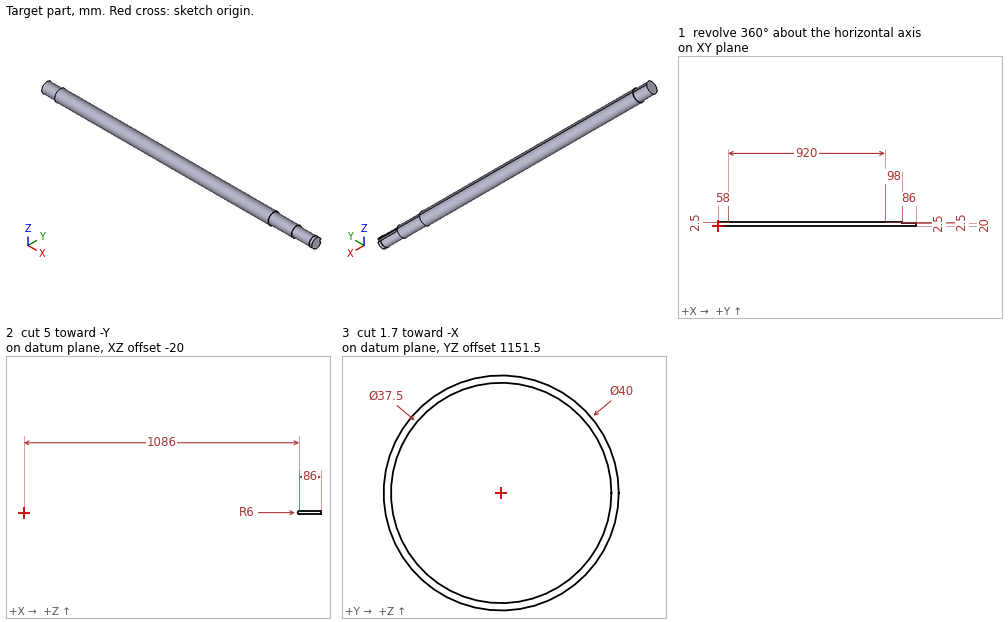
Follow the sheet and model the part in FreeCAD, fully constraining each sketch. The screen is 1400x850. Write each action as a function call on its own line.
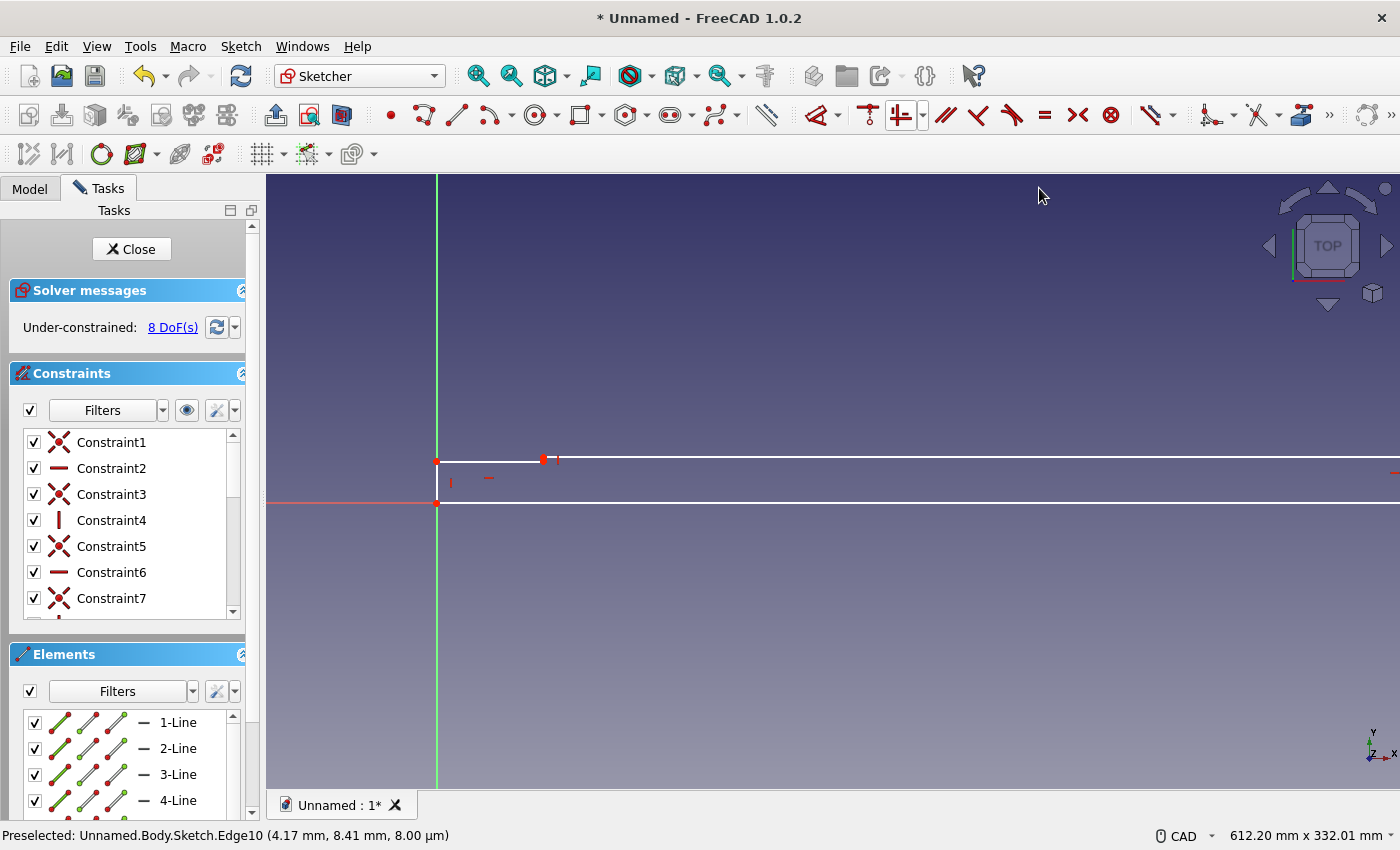
scroll(442, 482, down, 6)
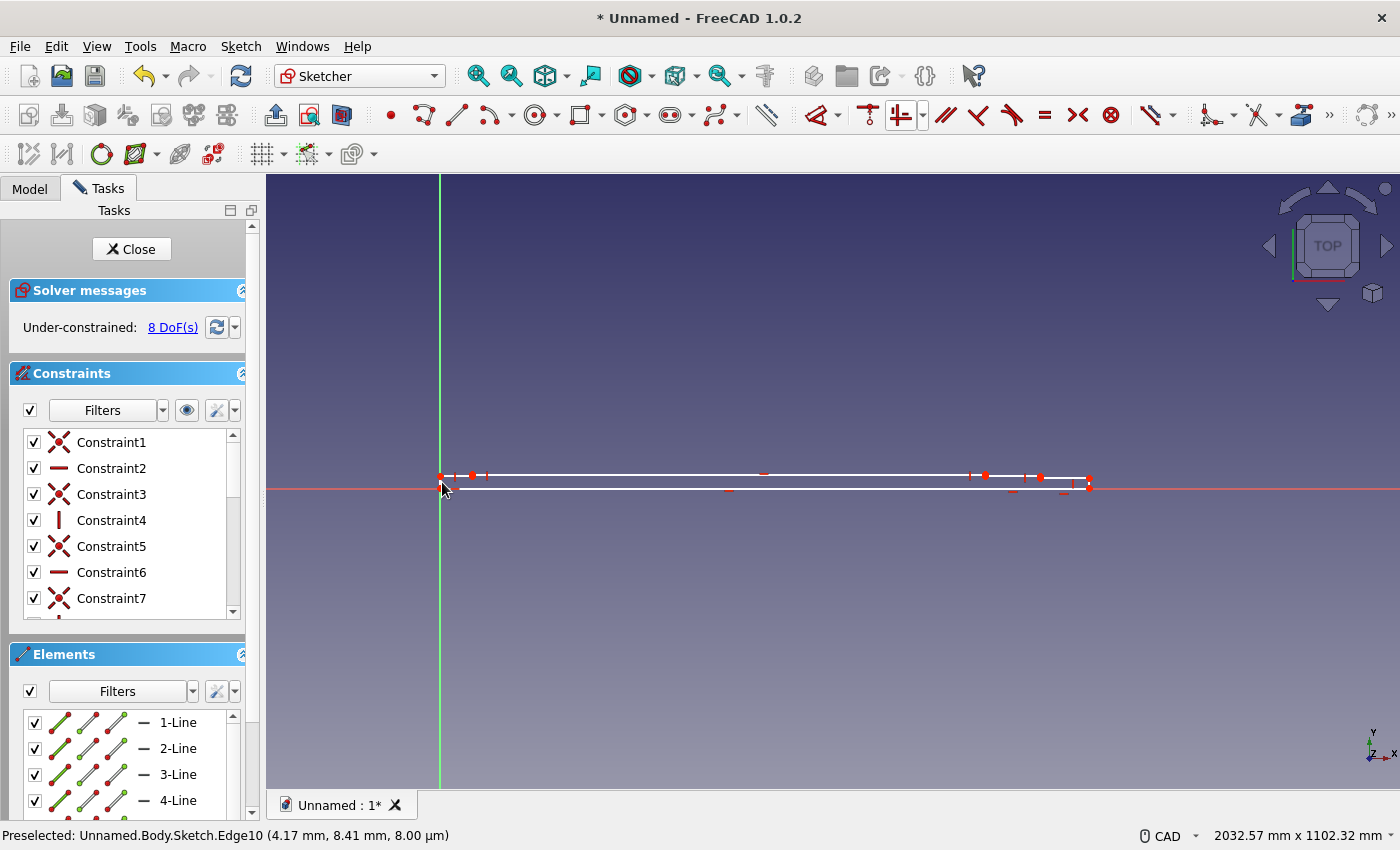
scroll(1089, 486, up, 8)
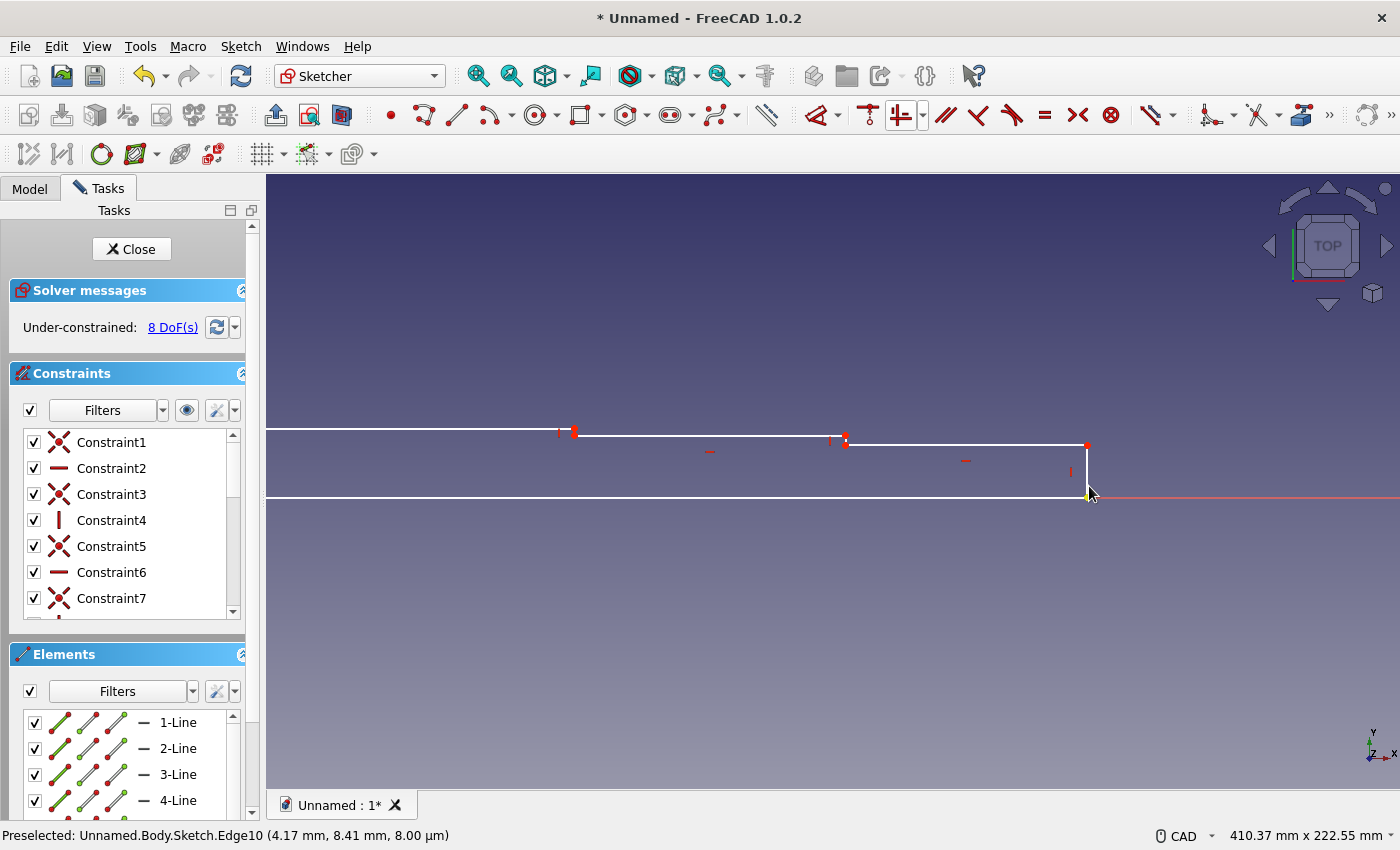
click(1087, 482)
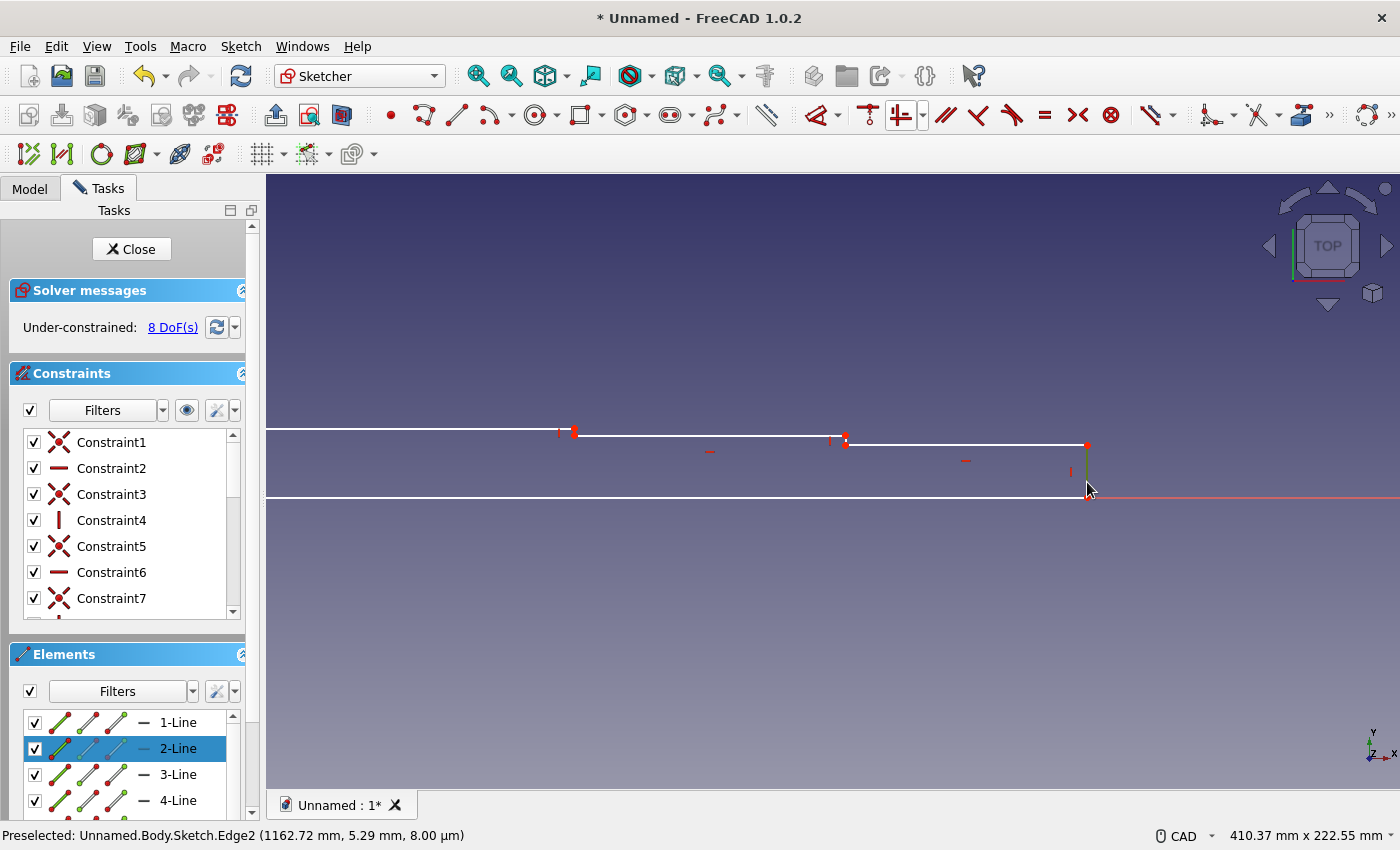
click(838, 116)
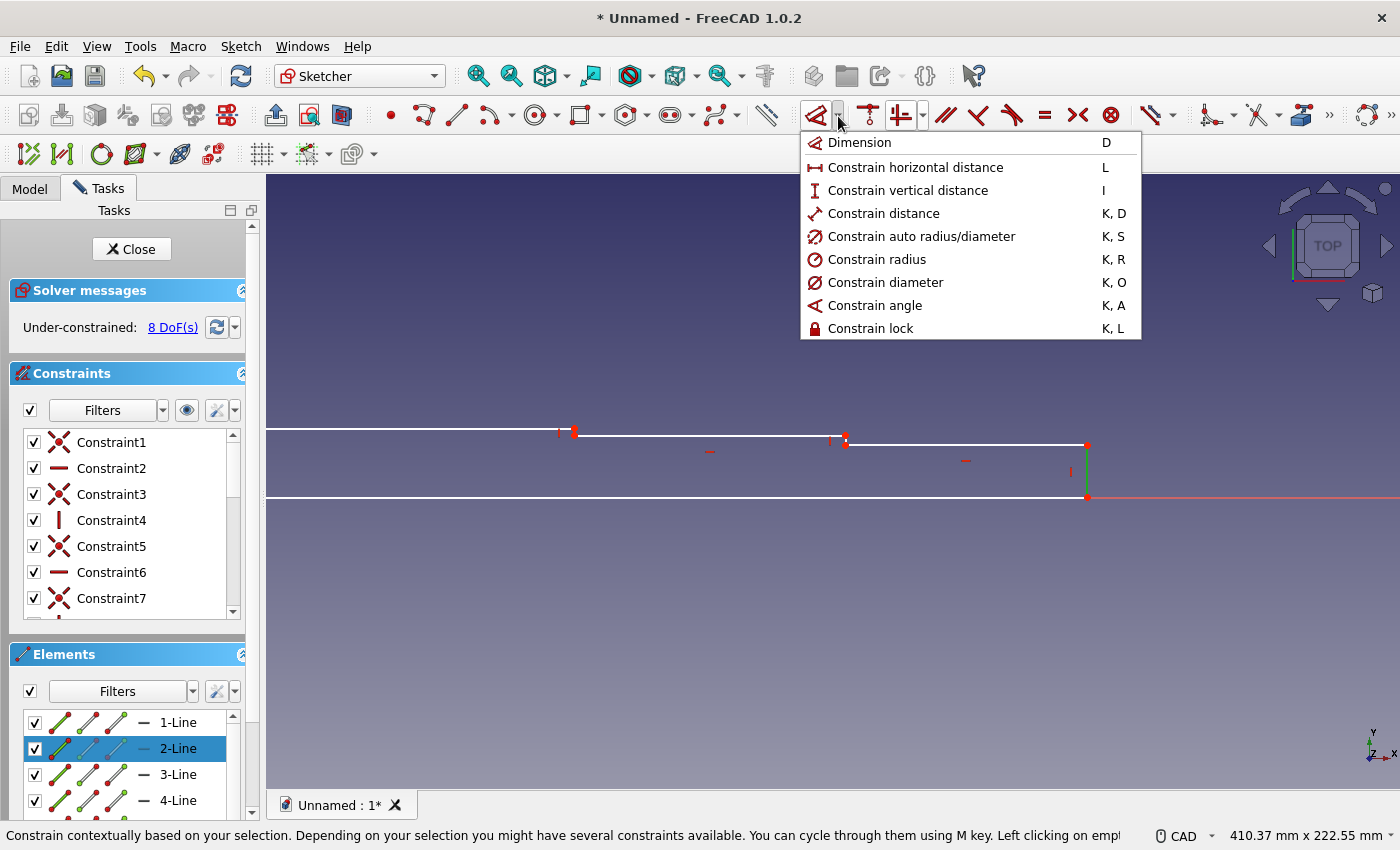
click(971, 190)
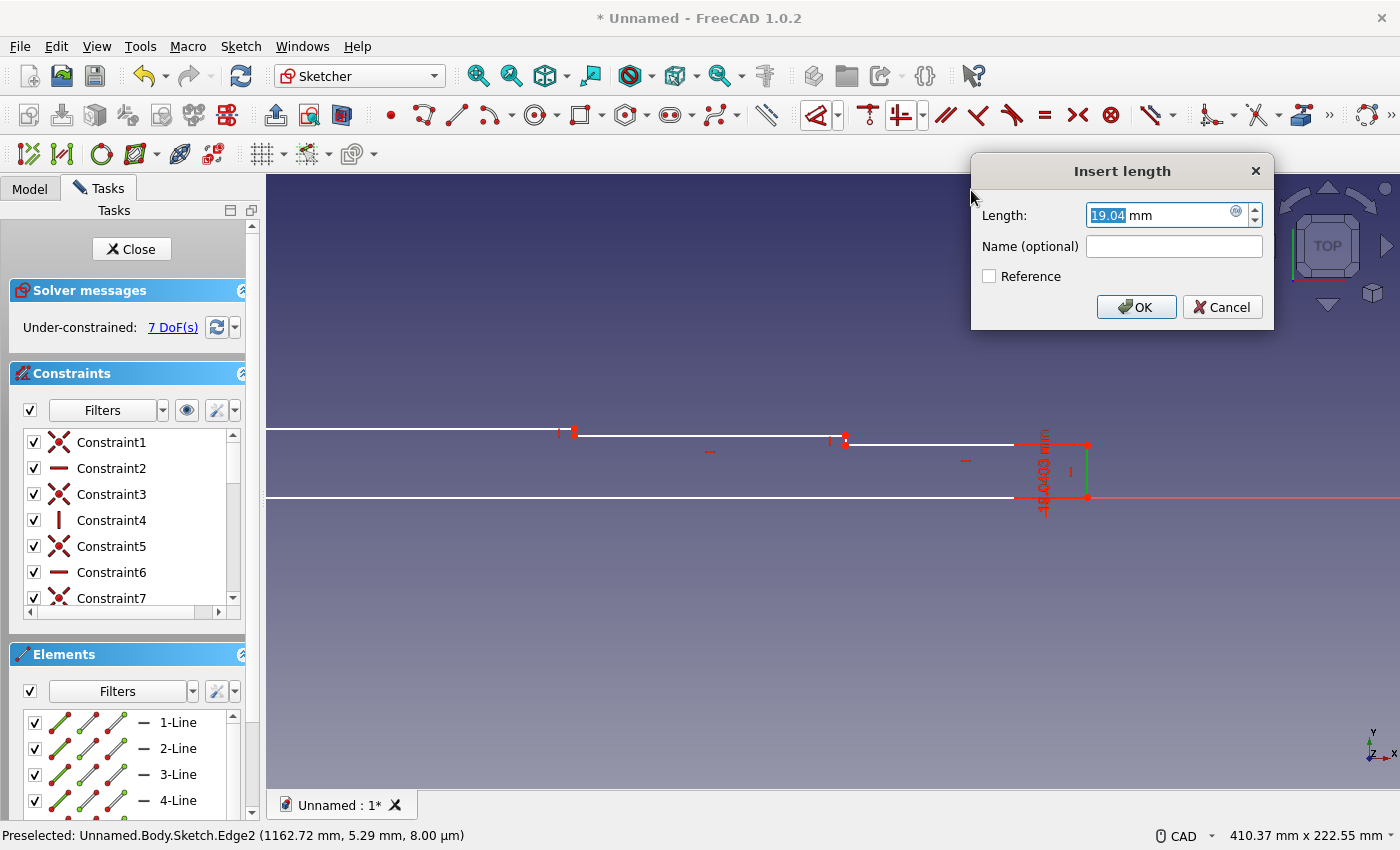
text(20)
key(Return)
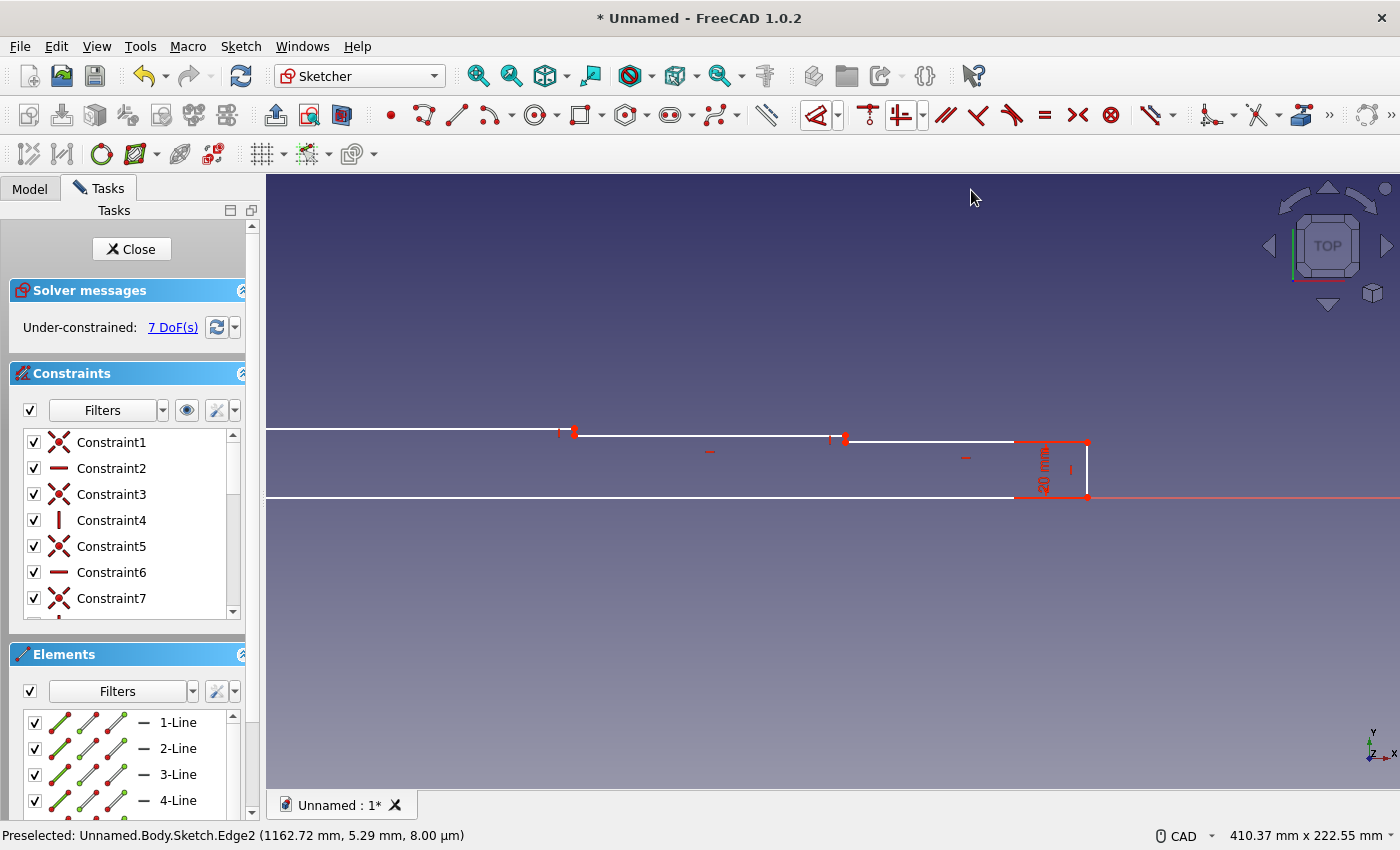
scroll(1090, 486, down, 8)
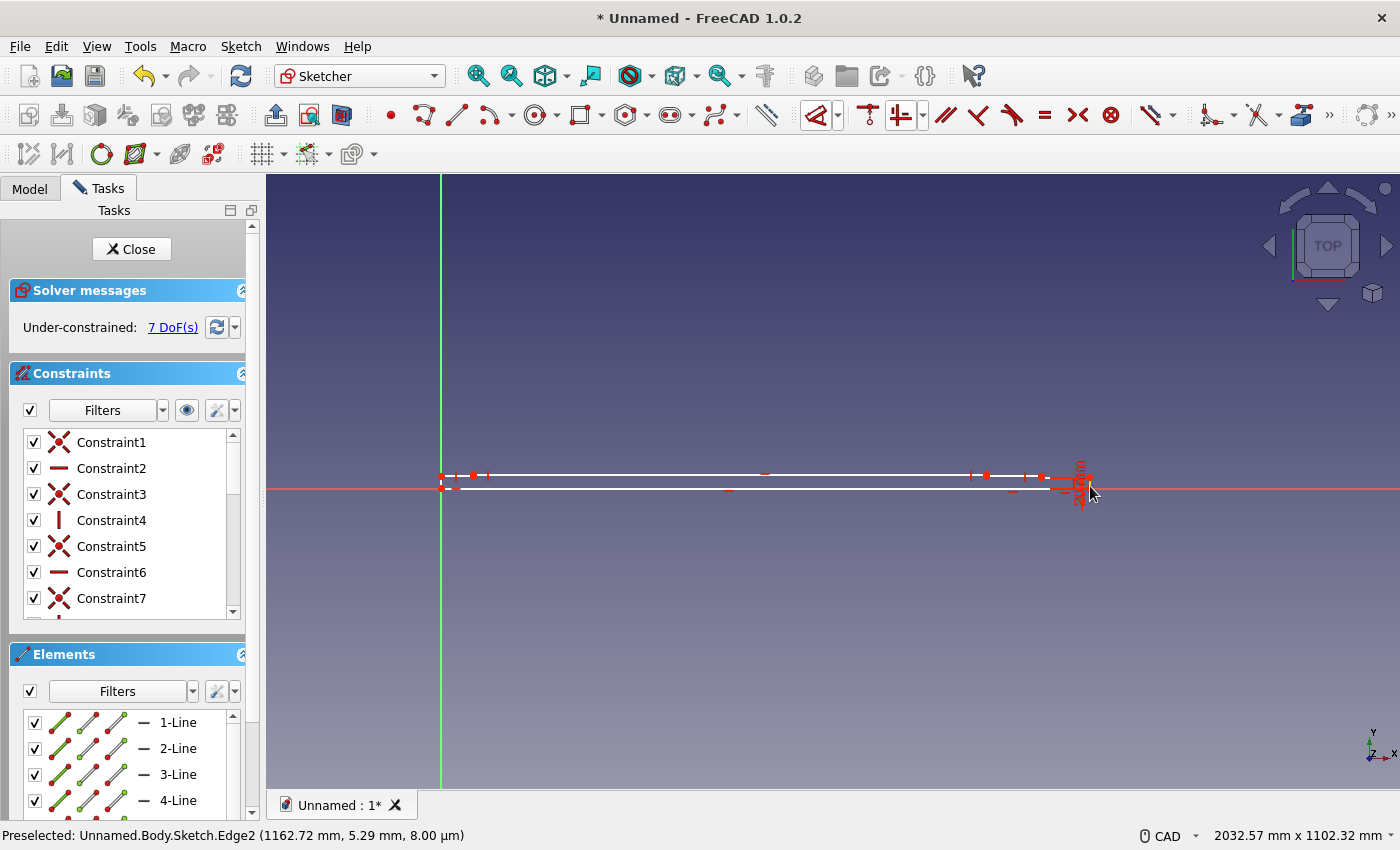
scroll(1075, 478, up, 2)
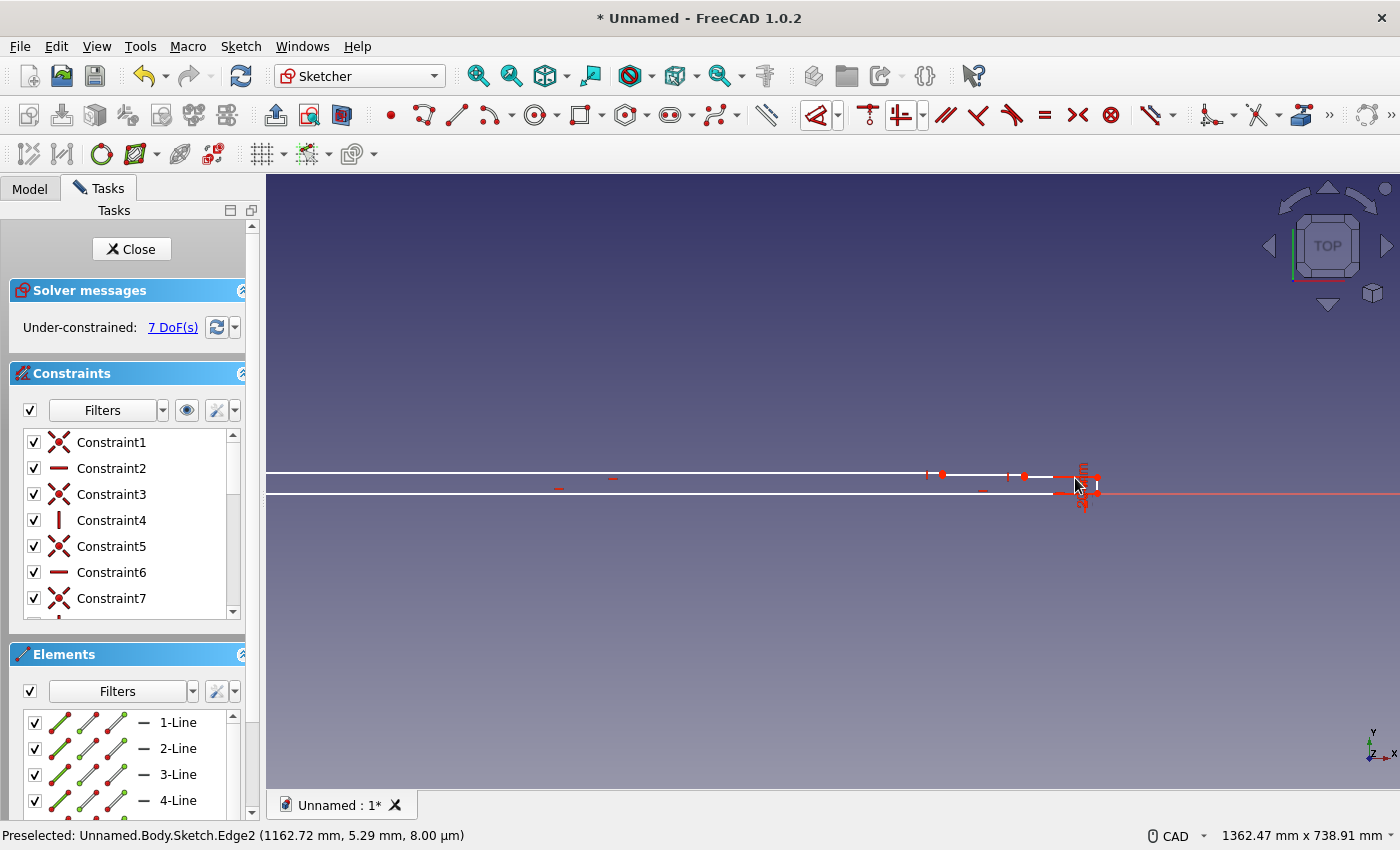
click(1075, 477)